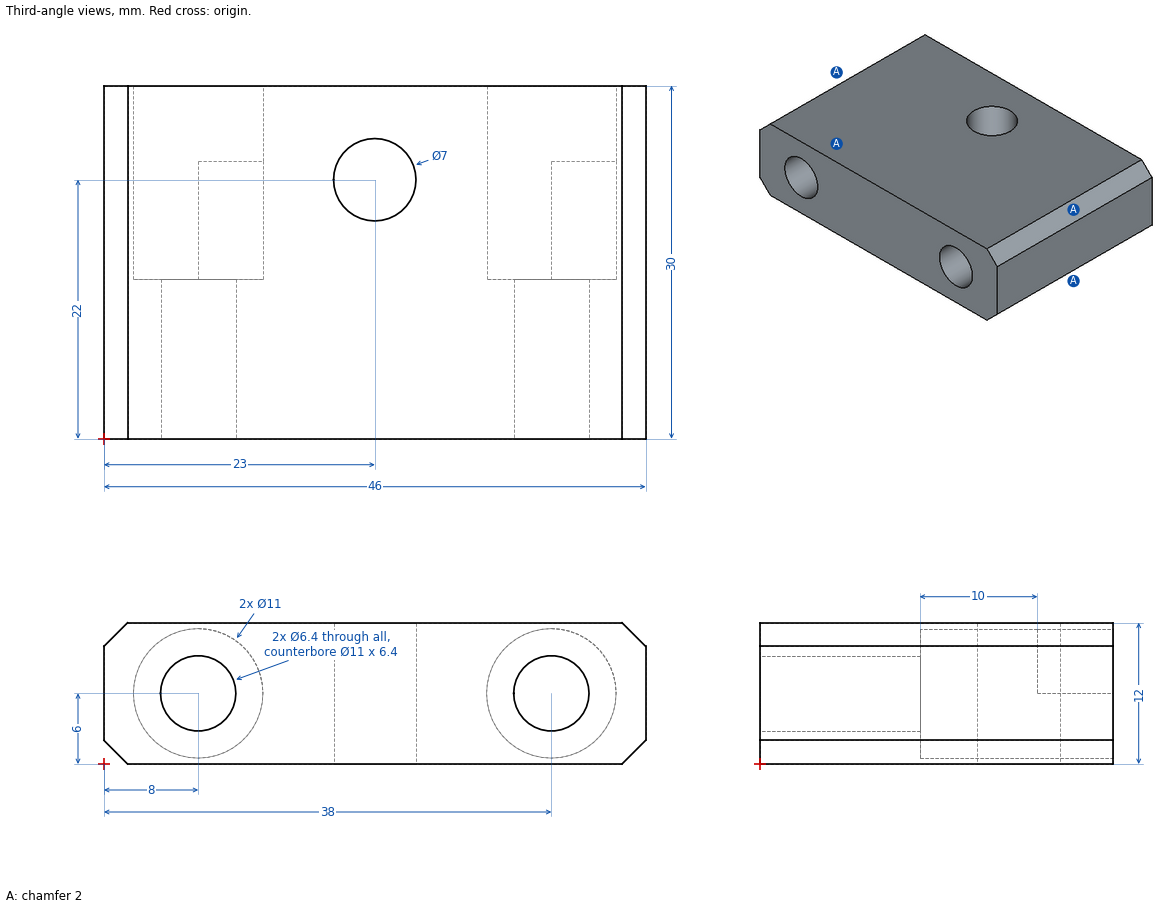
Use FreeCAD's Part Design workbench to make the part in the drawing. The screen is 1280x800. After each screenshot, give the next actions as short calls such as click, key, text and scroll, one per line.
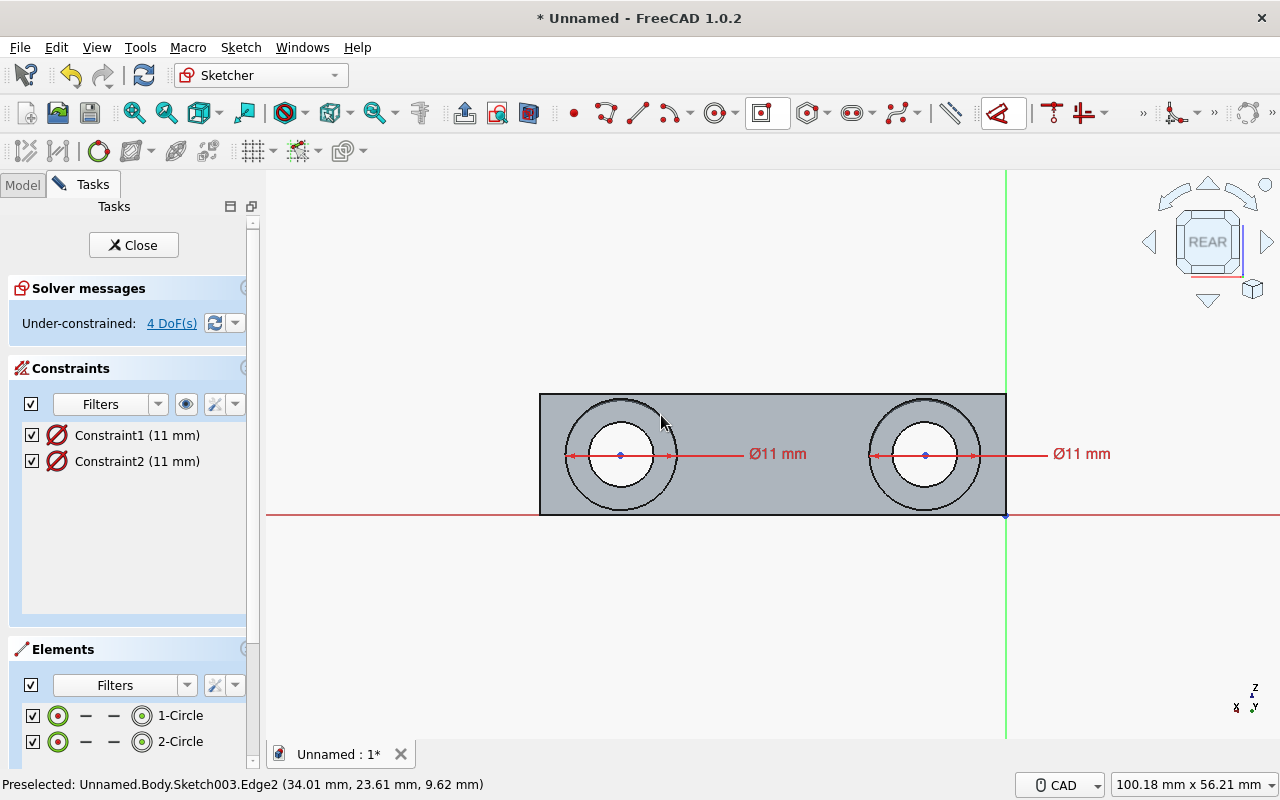
click(925, 456)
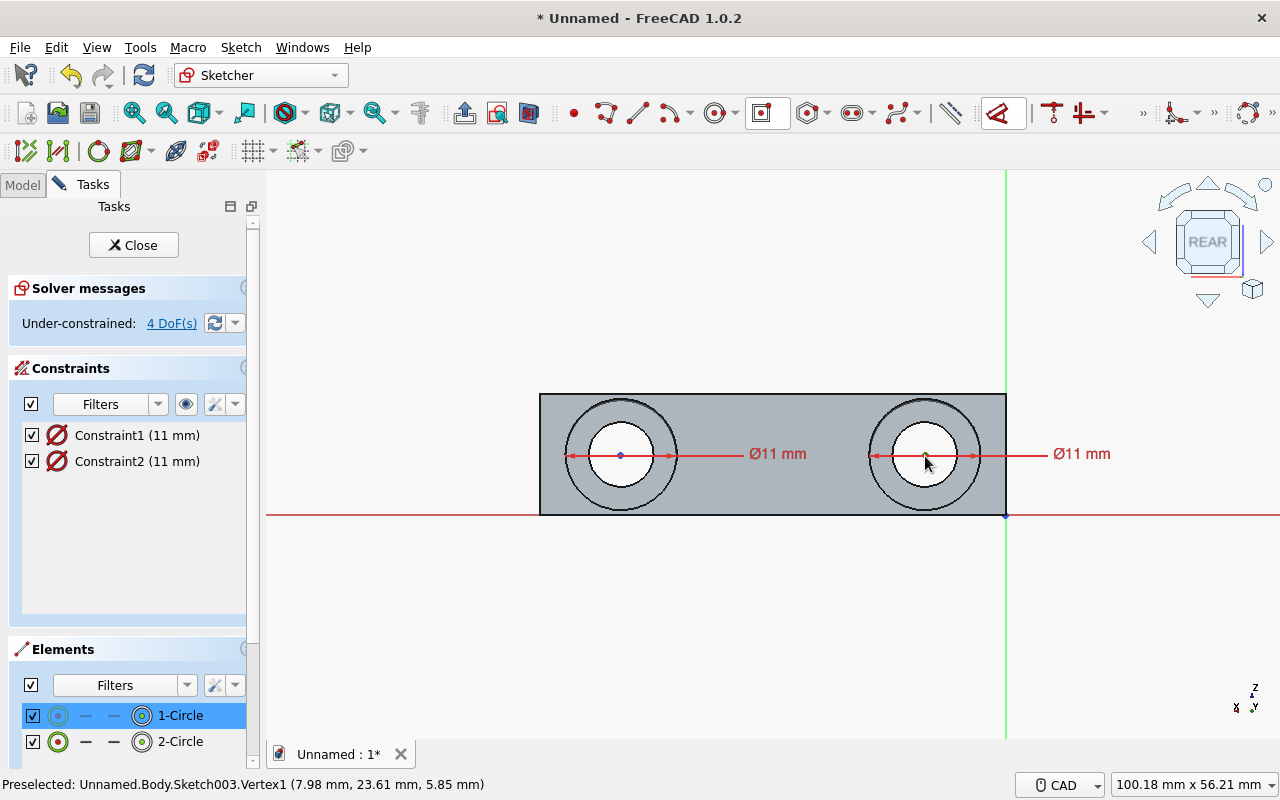
click(621, 456)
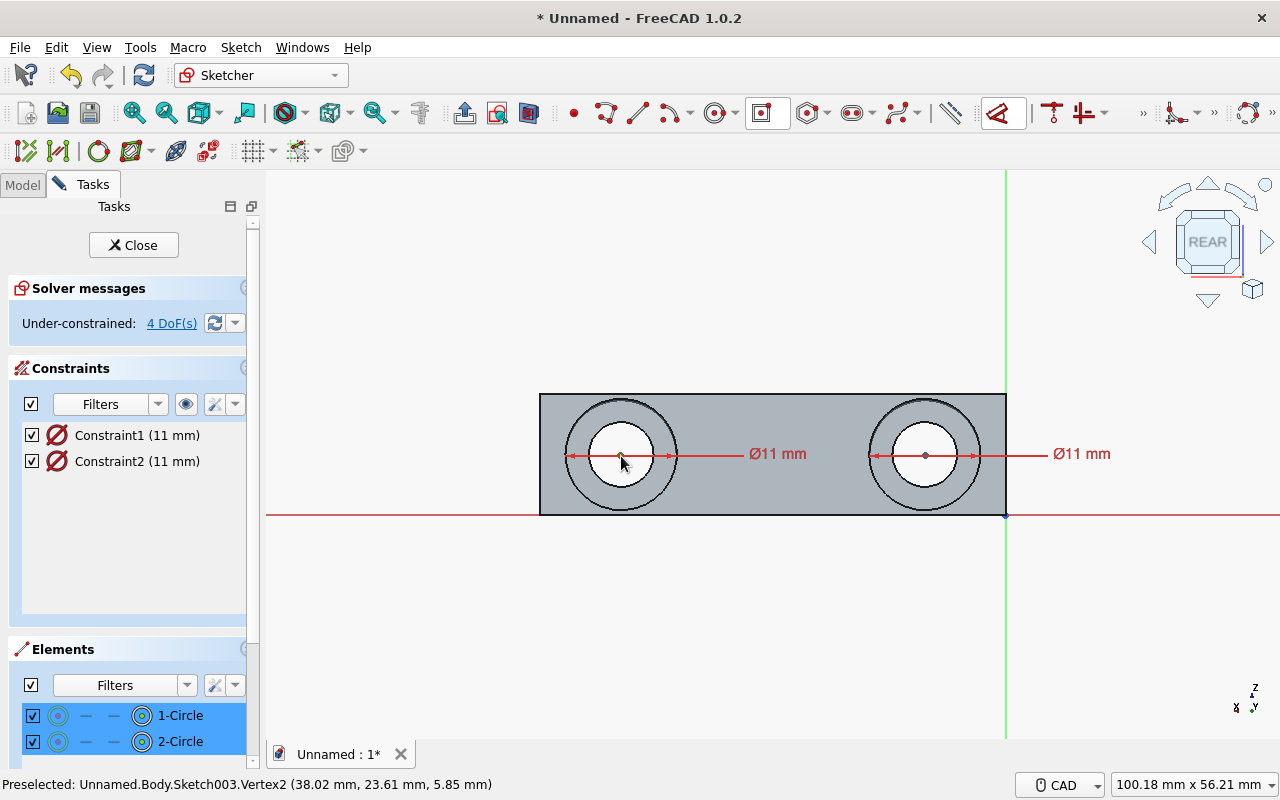
key(h)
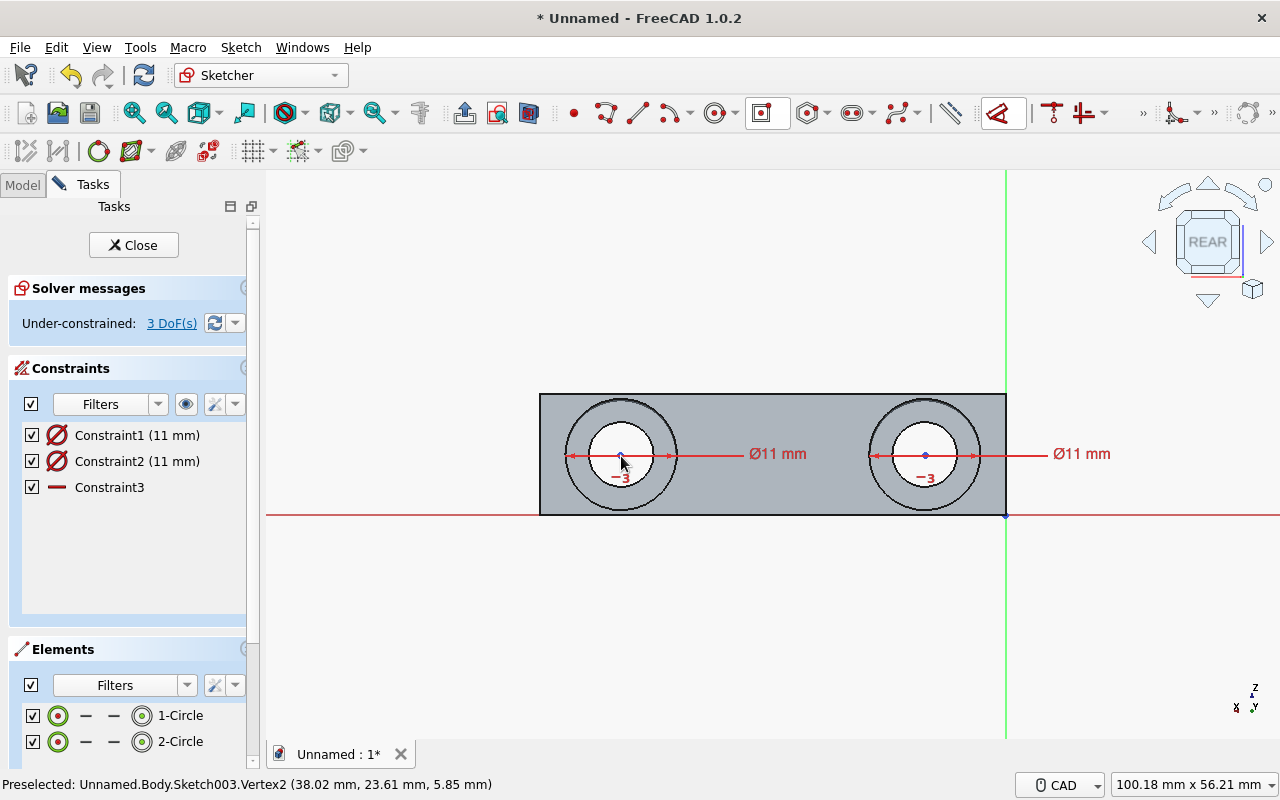
click(925, 456)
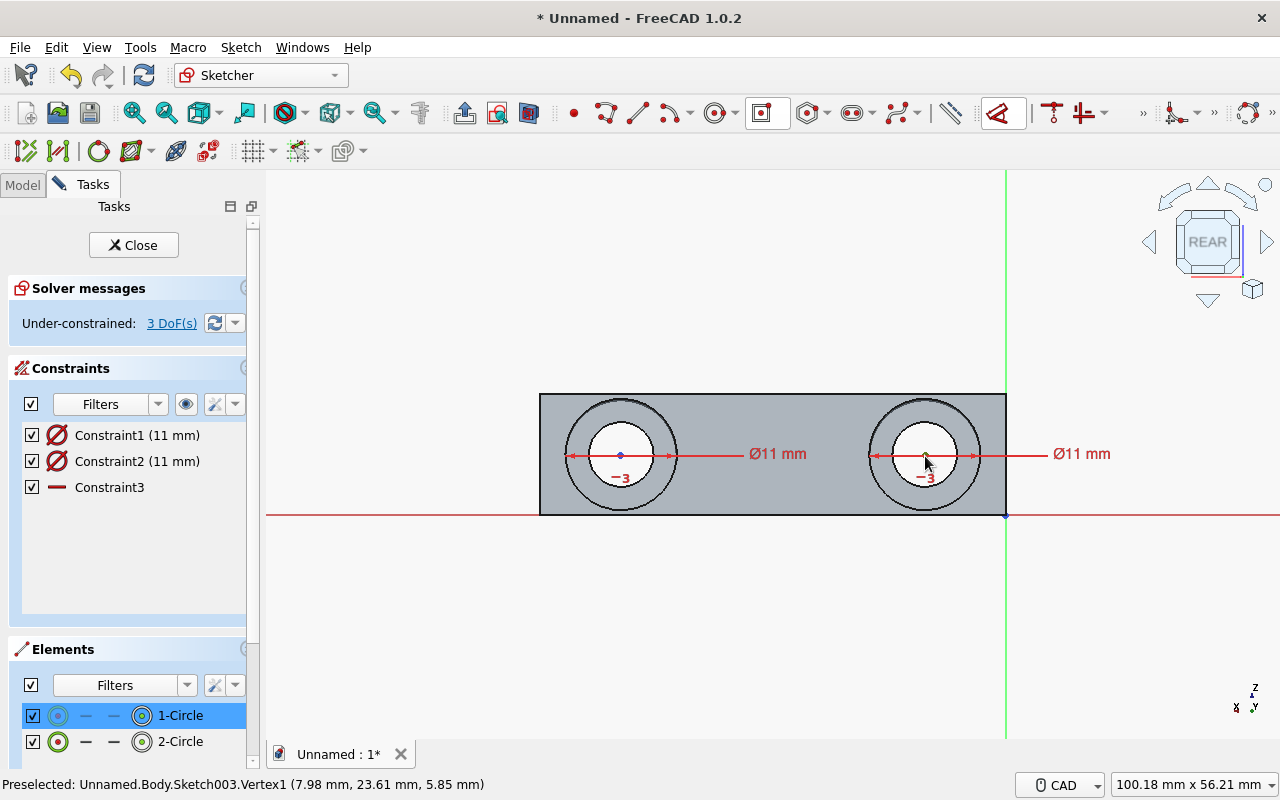
click(1020, 114)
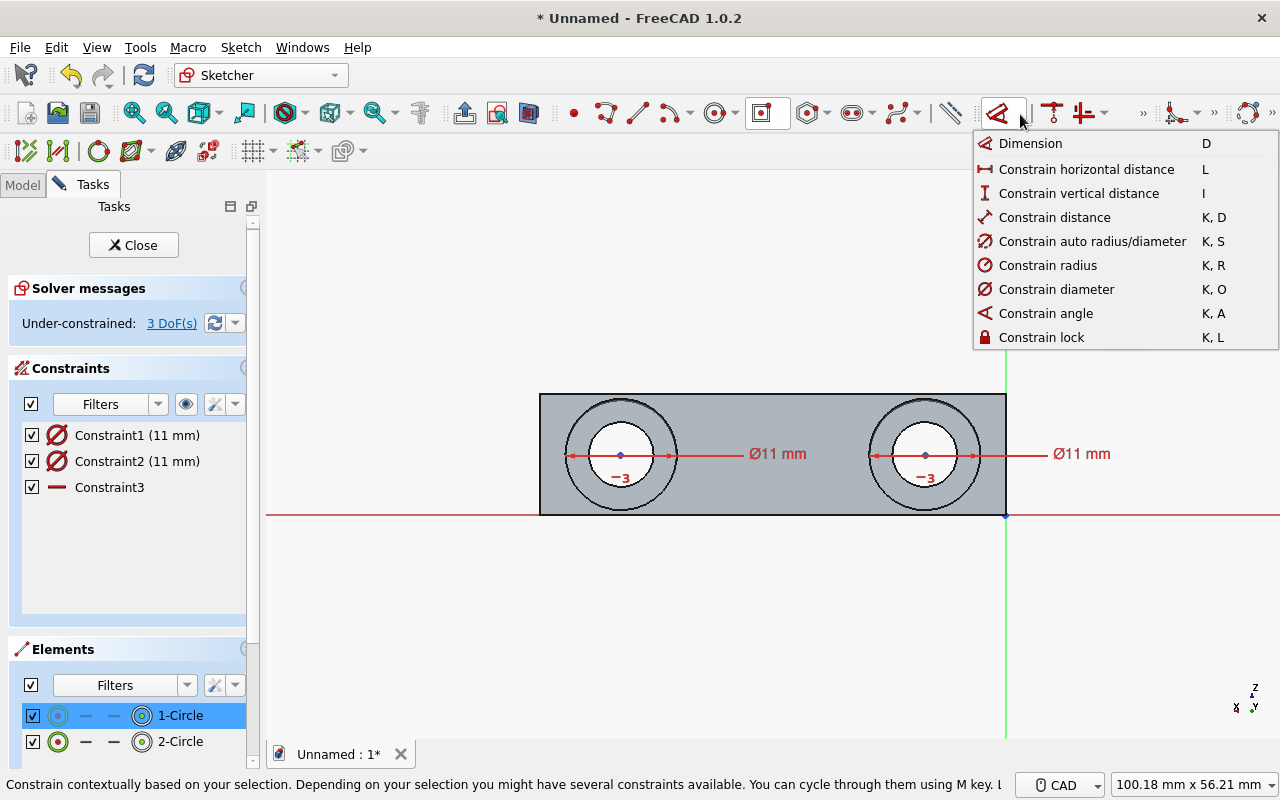
click(1126, 169)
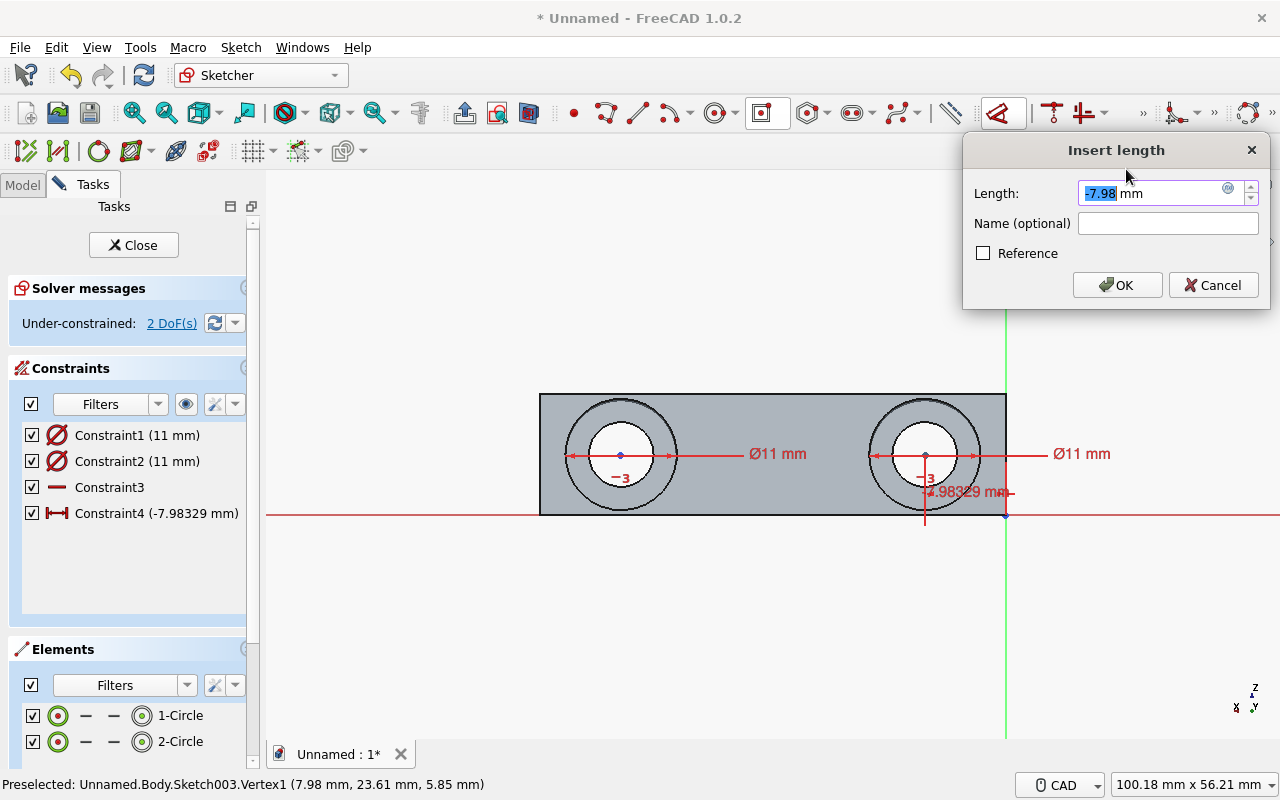
text(-8)
key(Return)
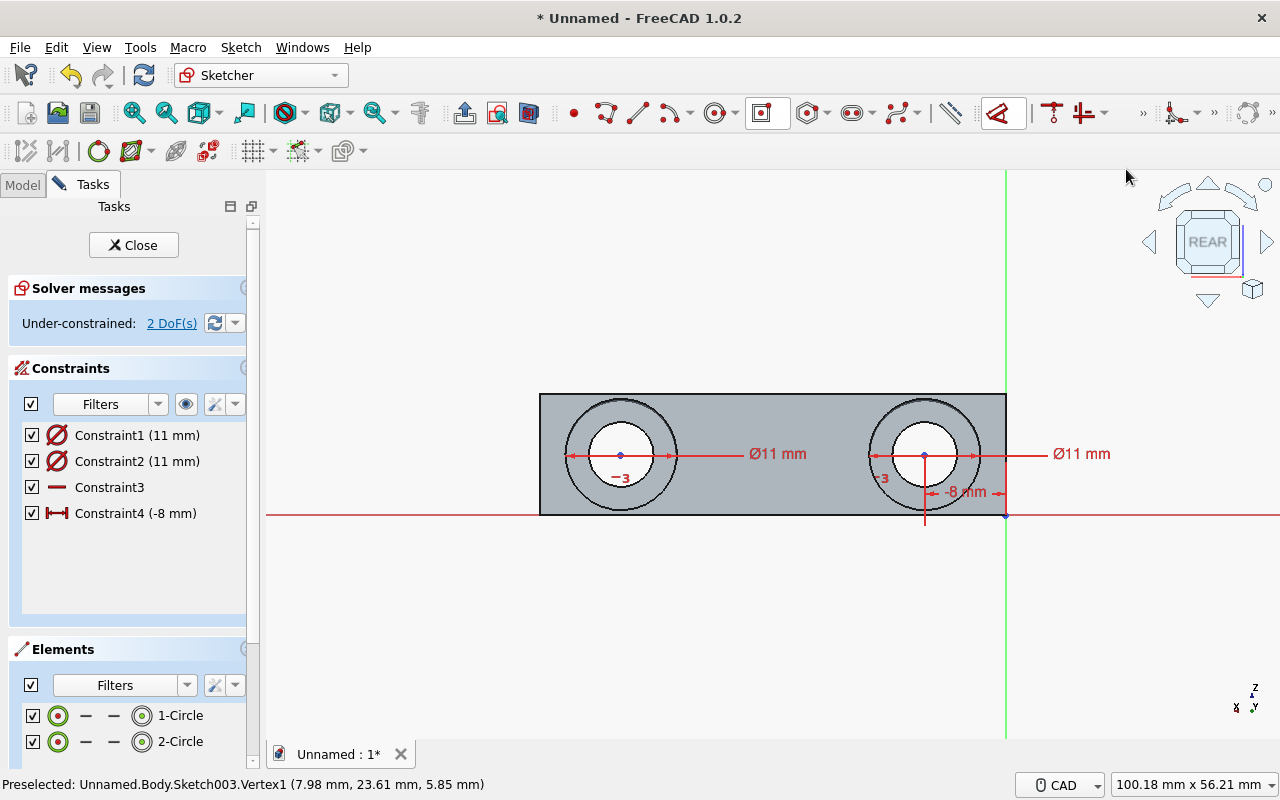
click(925, 456)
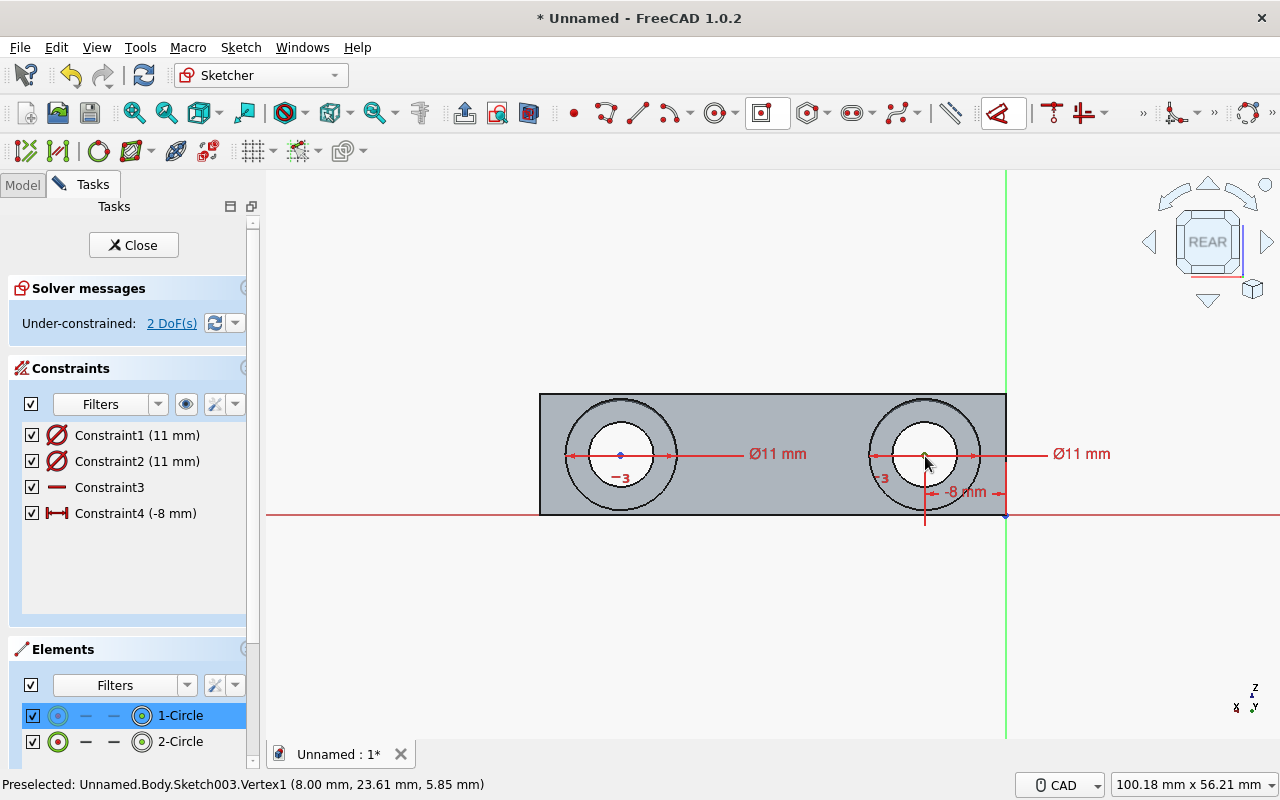
key(i)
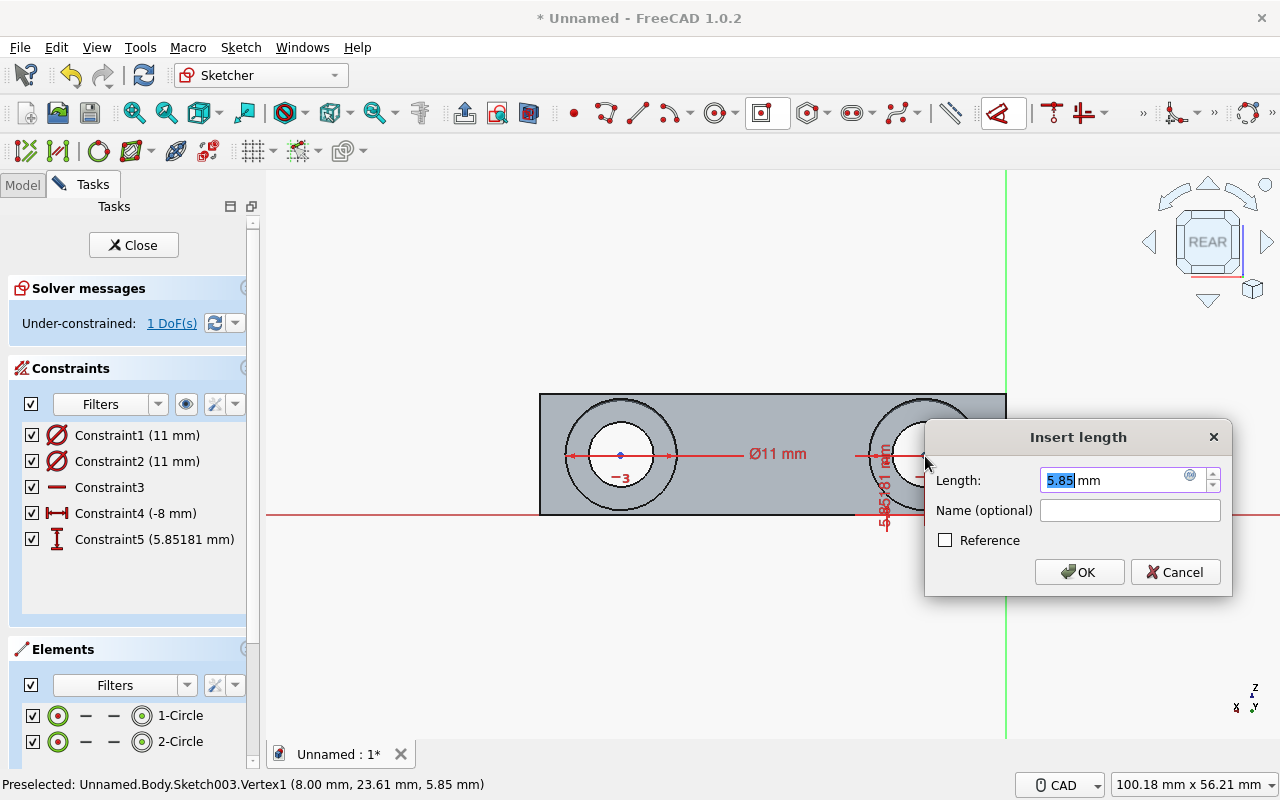
text(6)
key(Return)